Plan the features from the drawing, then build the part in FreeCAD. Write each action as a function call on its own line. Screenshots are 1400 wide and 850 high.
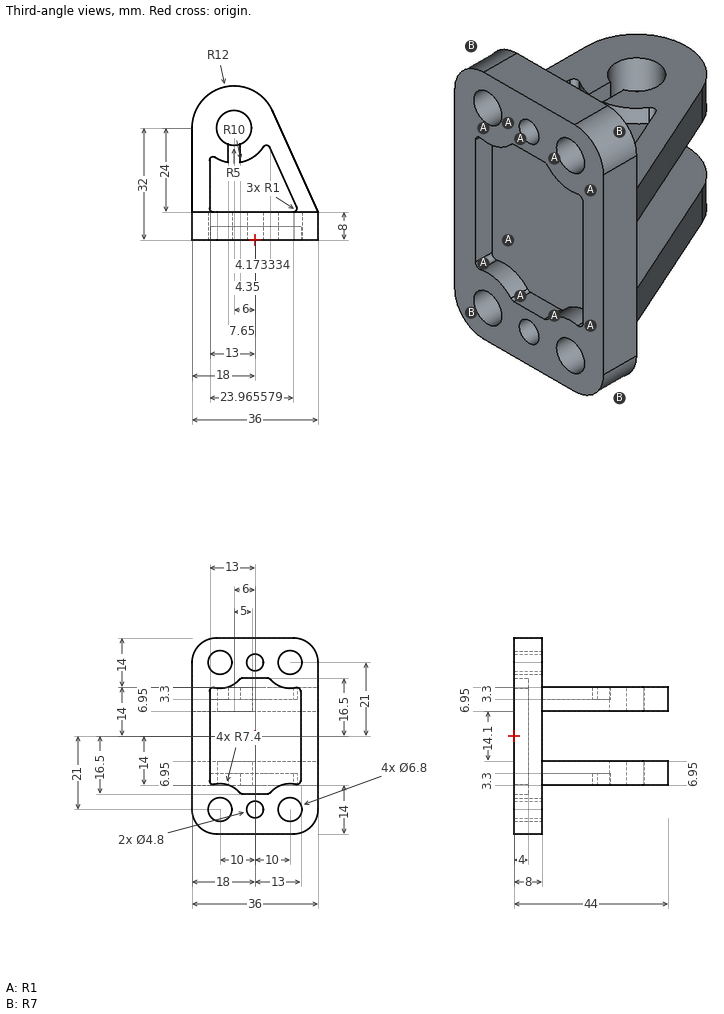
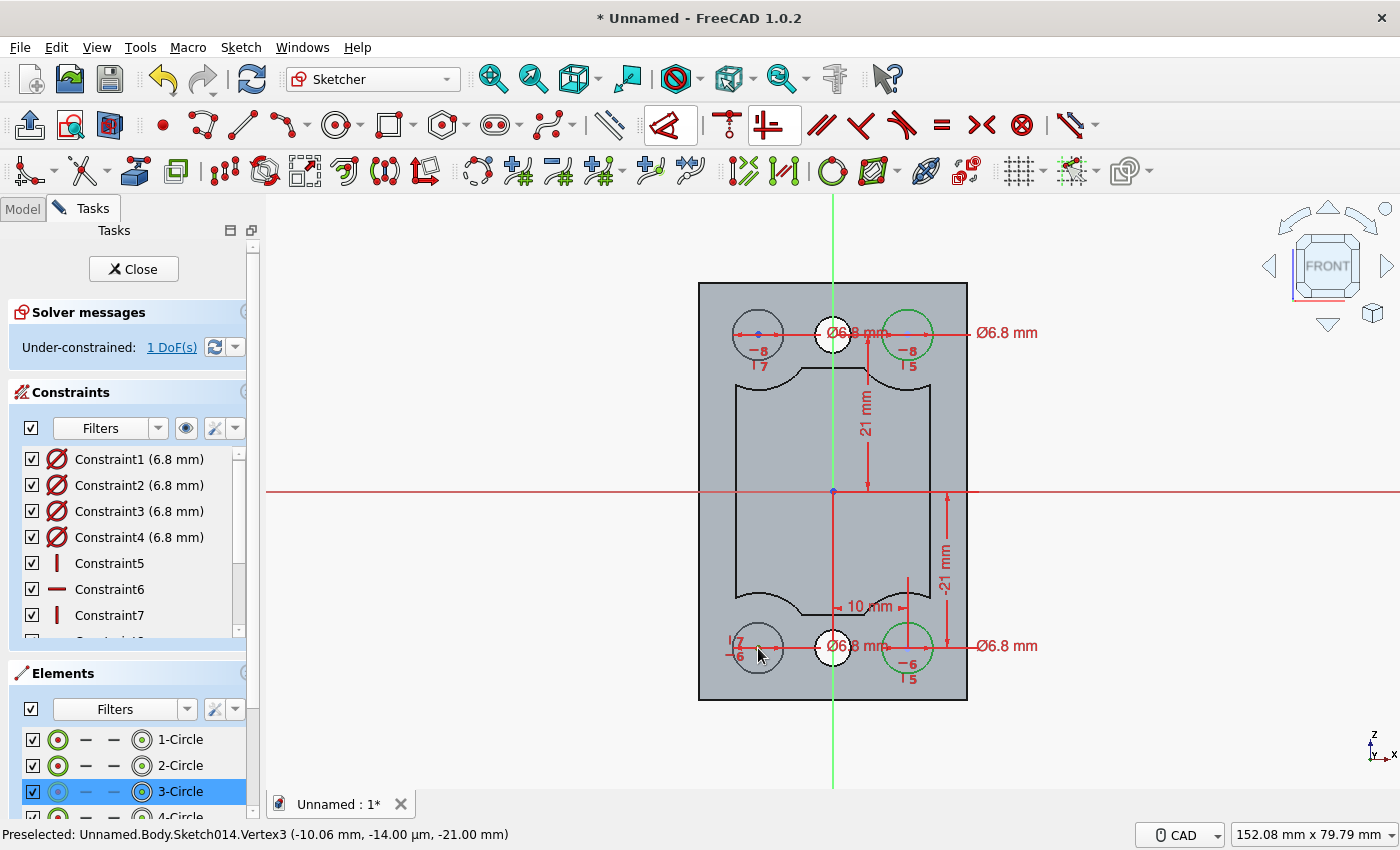
key(l)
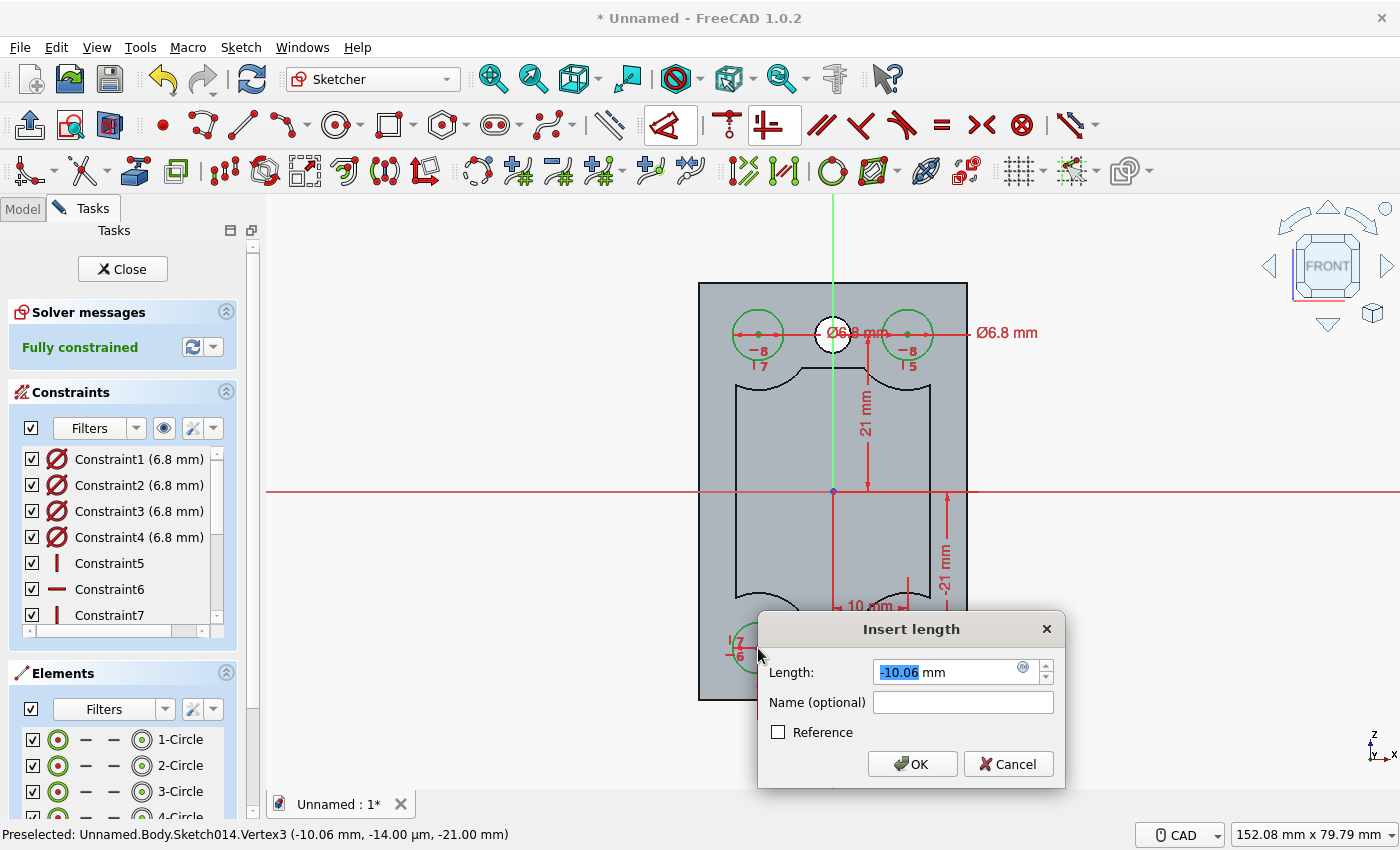
text(-10)
key(Return)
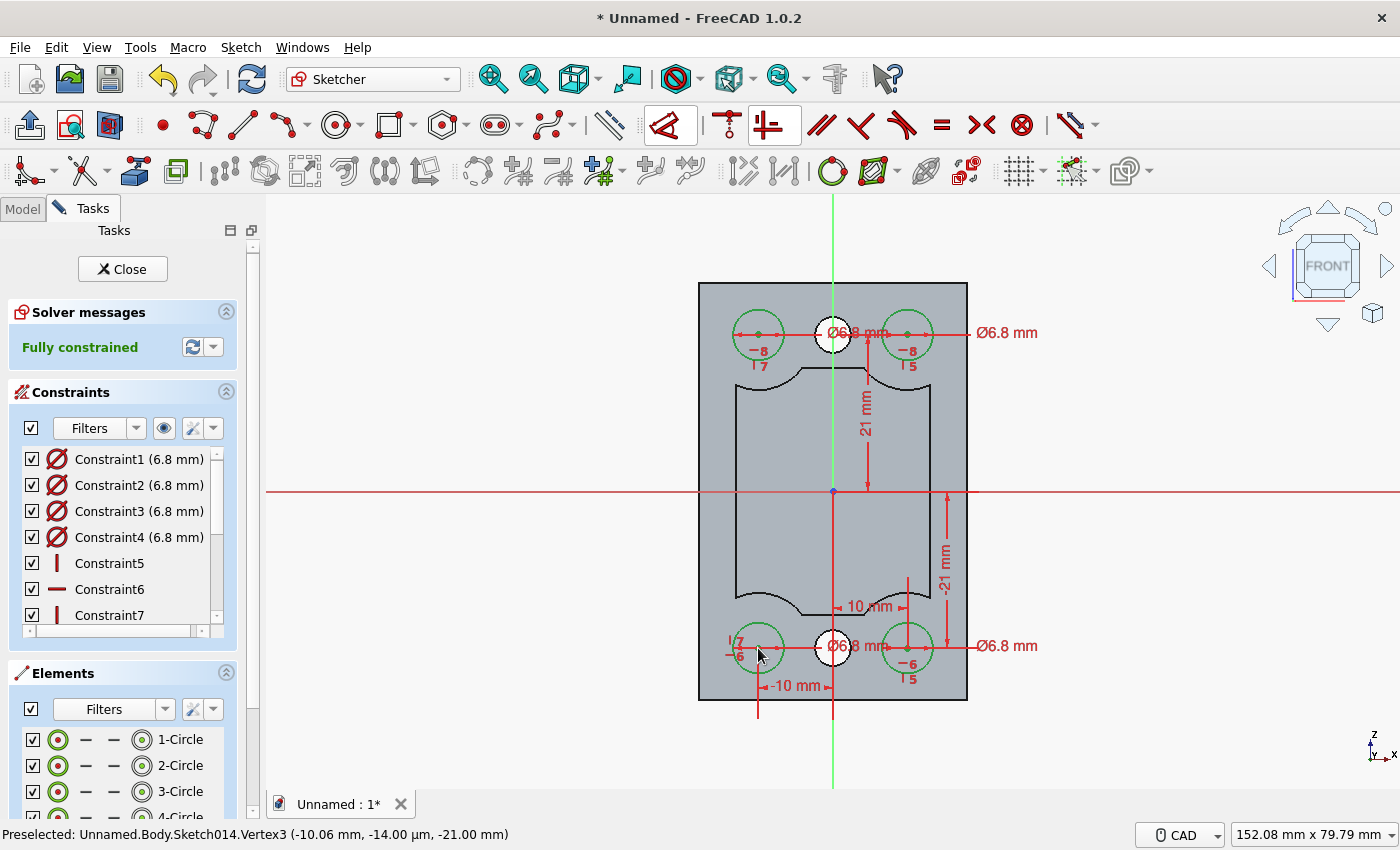
click(123, 269)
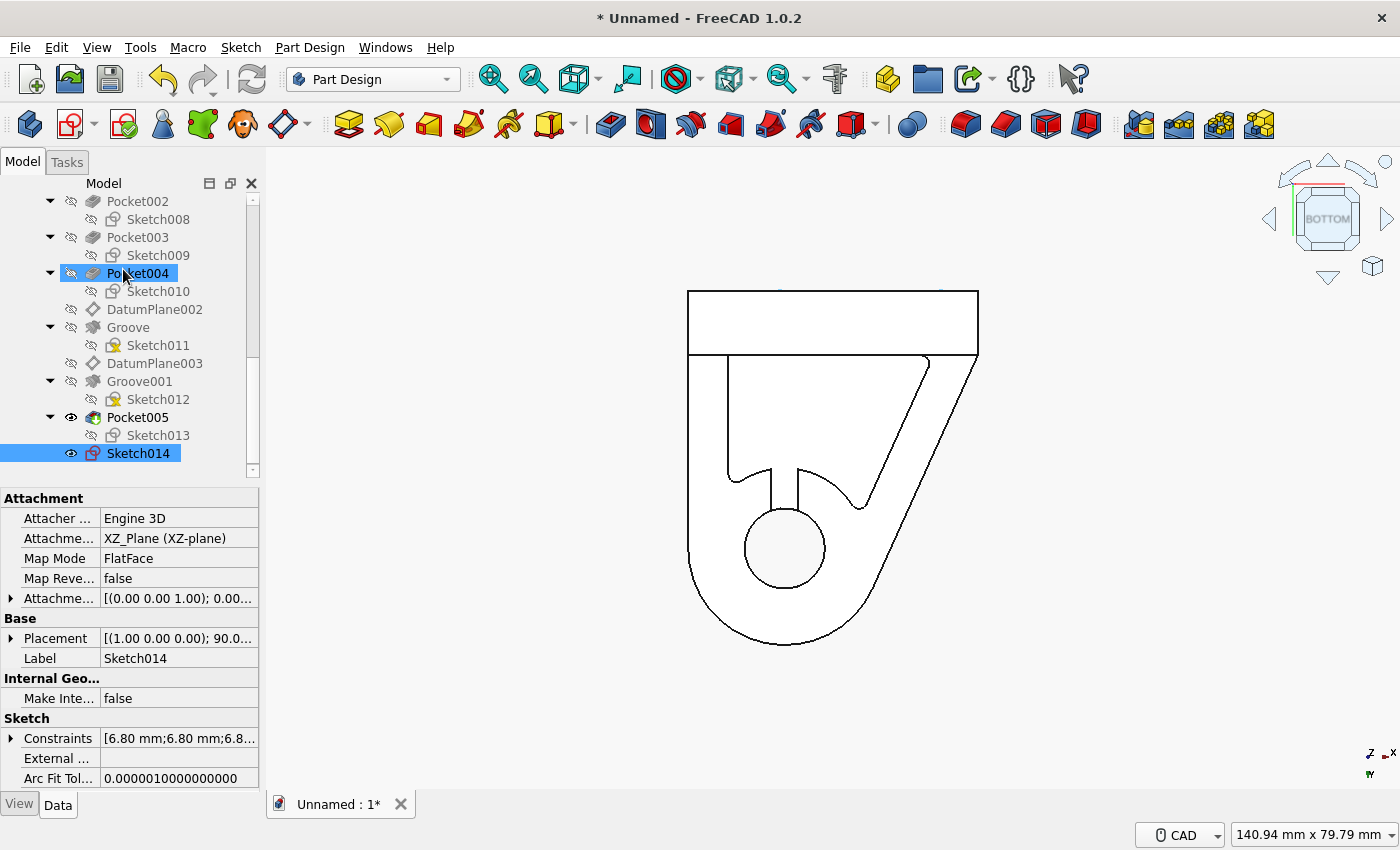
click(612, 124)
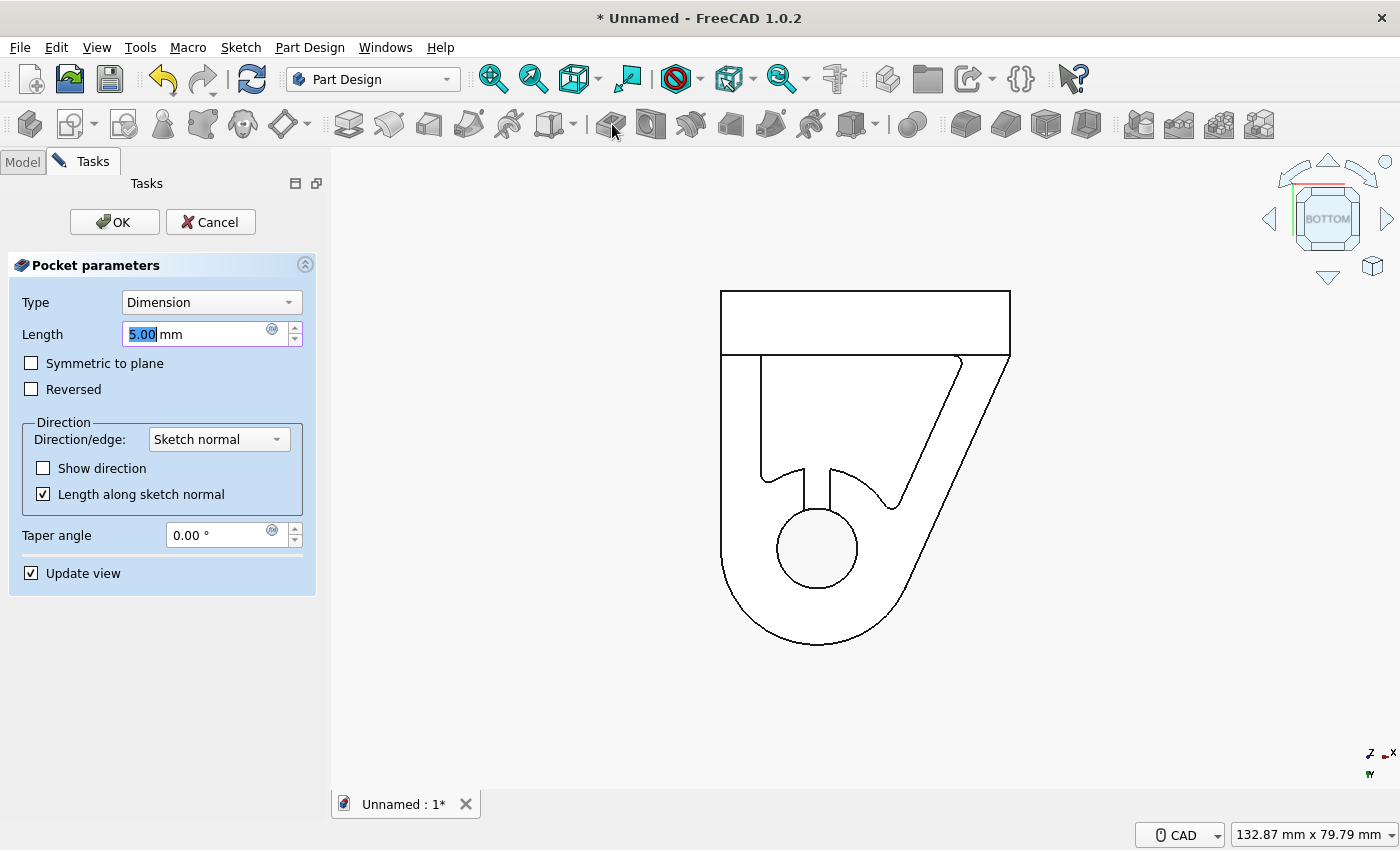
text(44)
key(Tab)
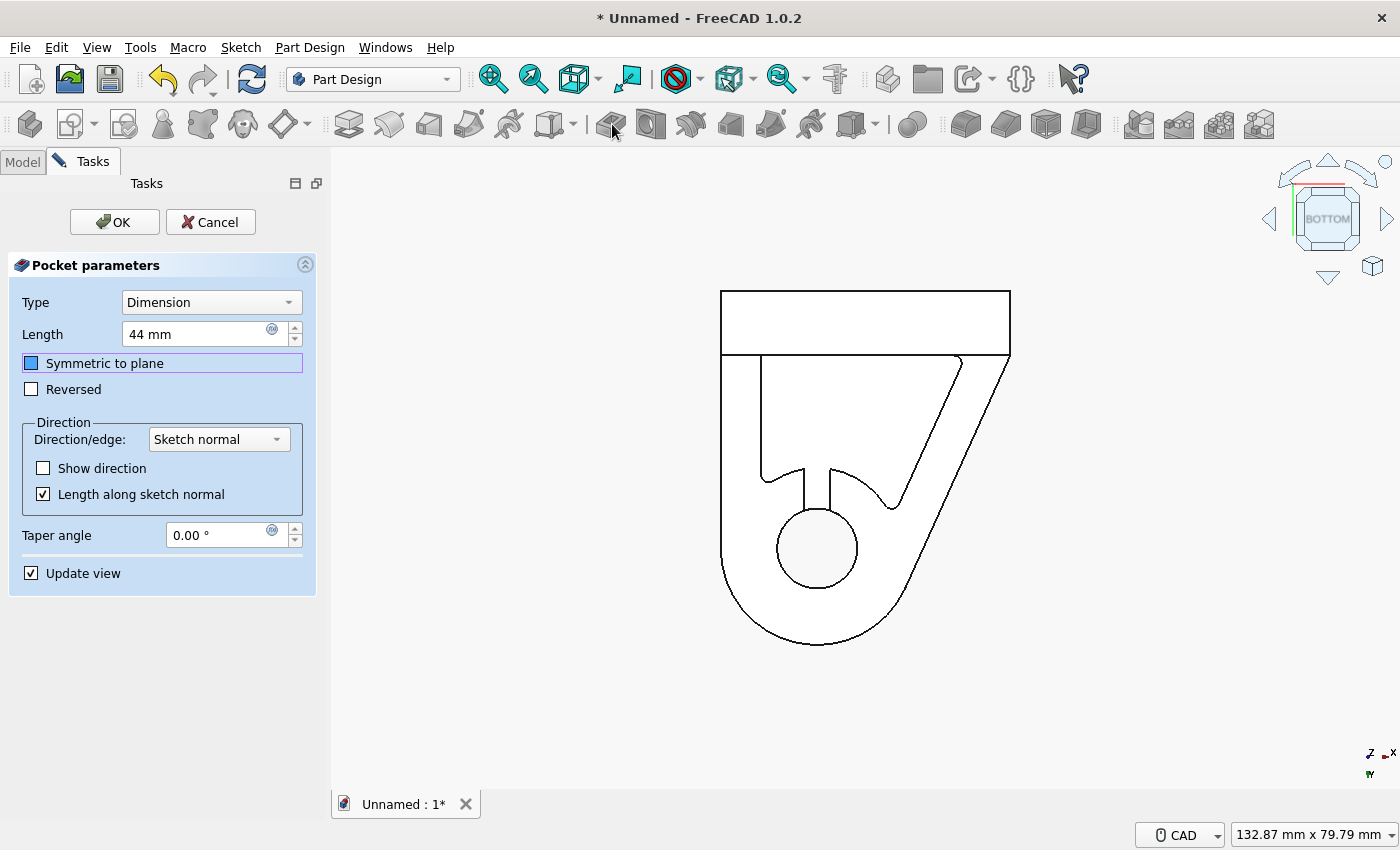
click(115, 222)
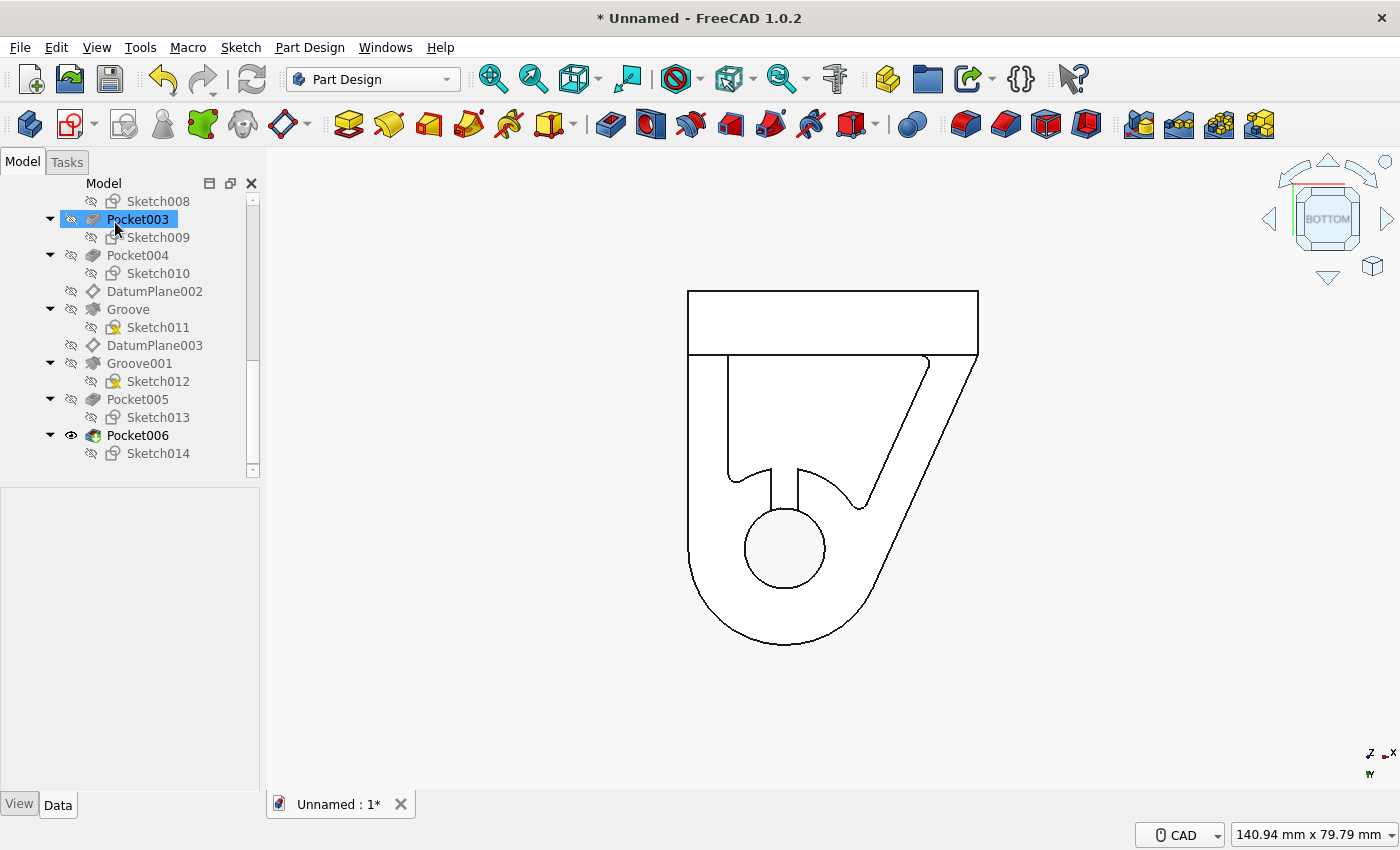
key(0)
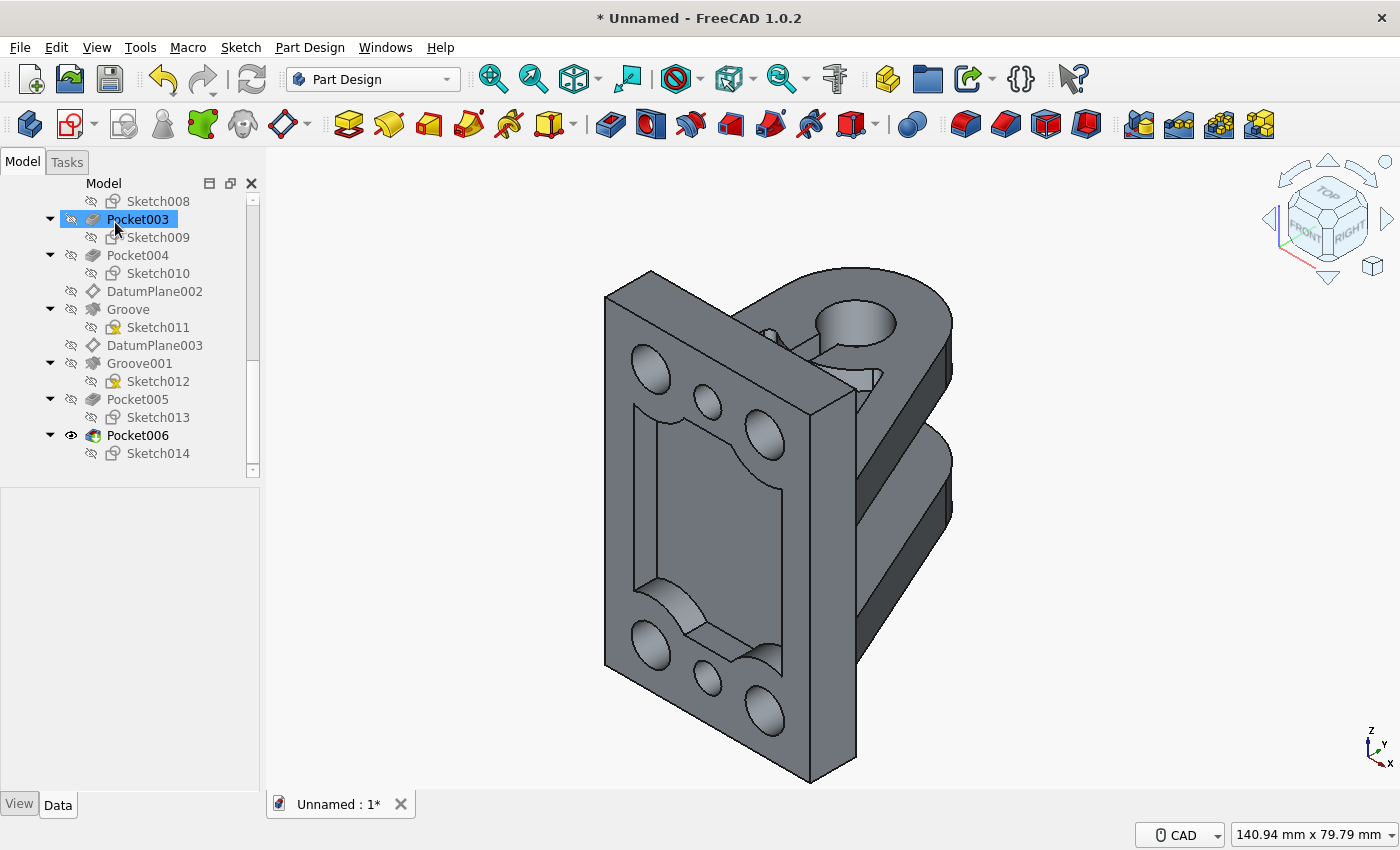
key(2)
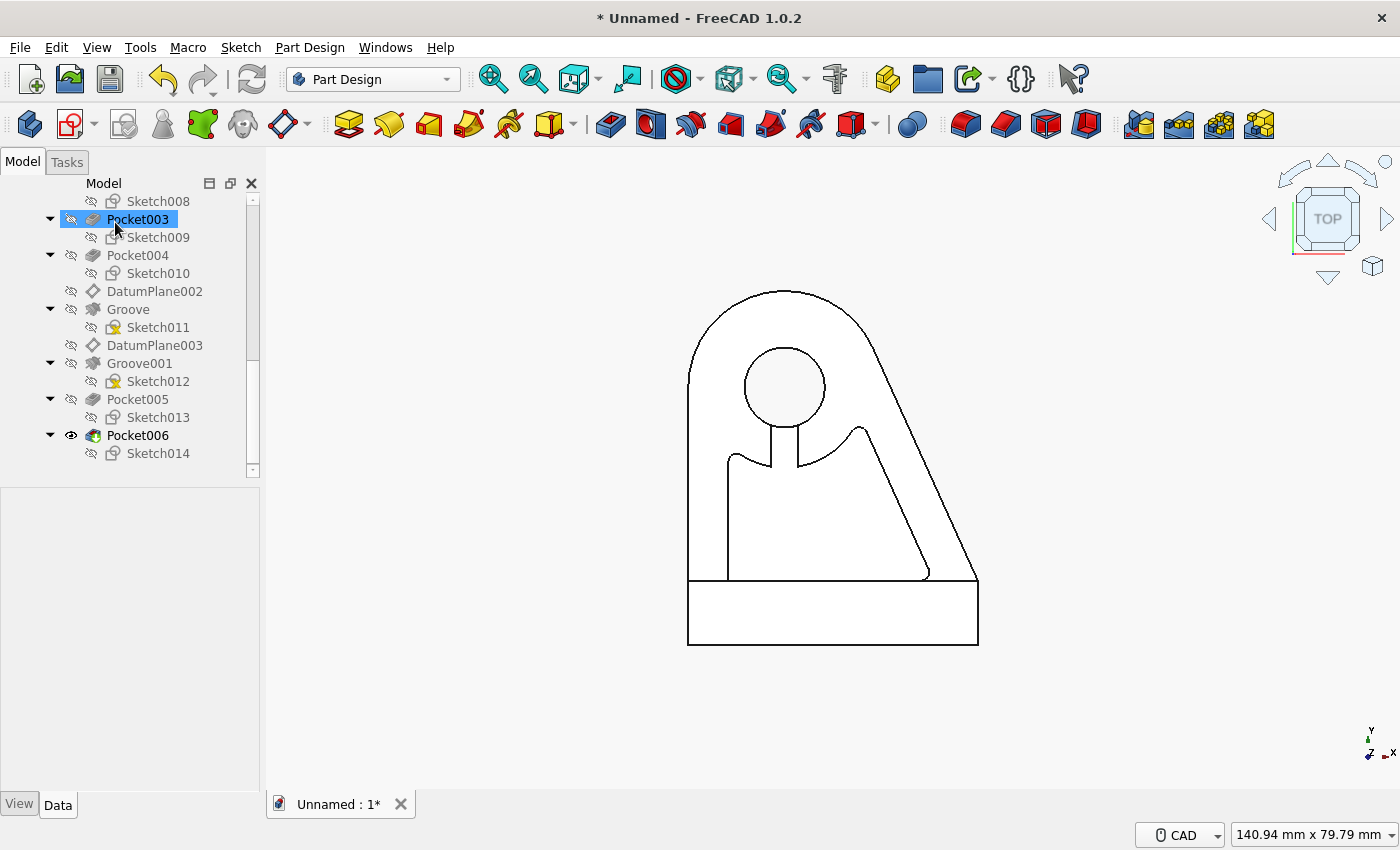
key(1)